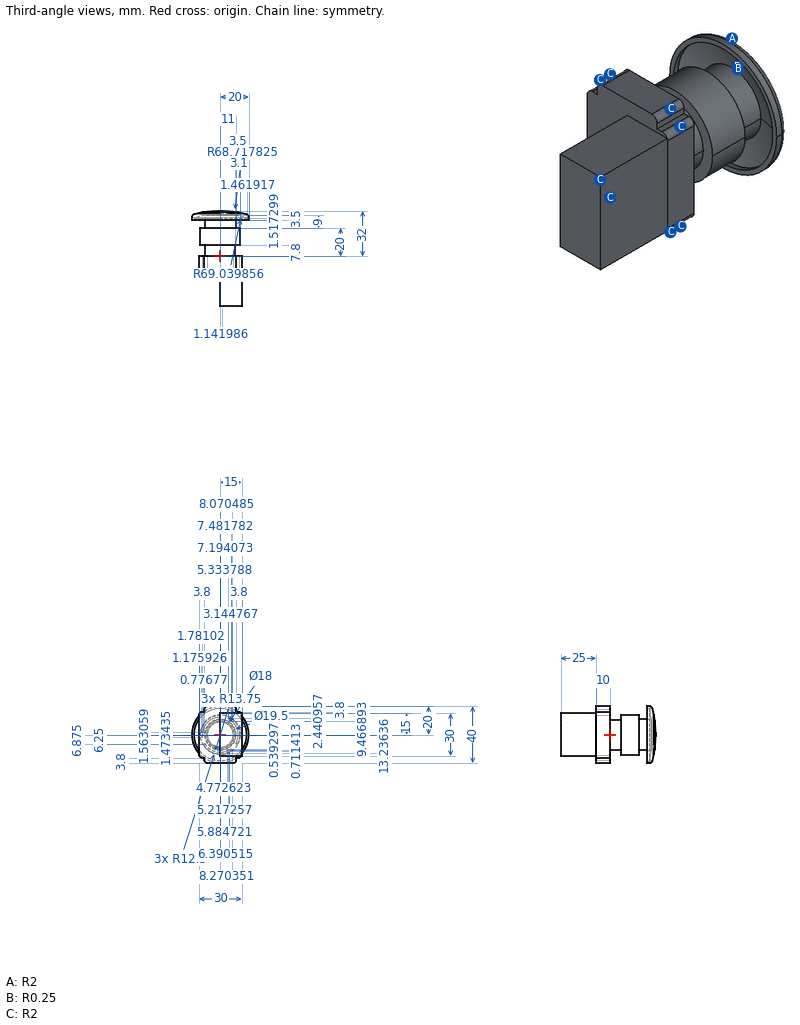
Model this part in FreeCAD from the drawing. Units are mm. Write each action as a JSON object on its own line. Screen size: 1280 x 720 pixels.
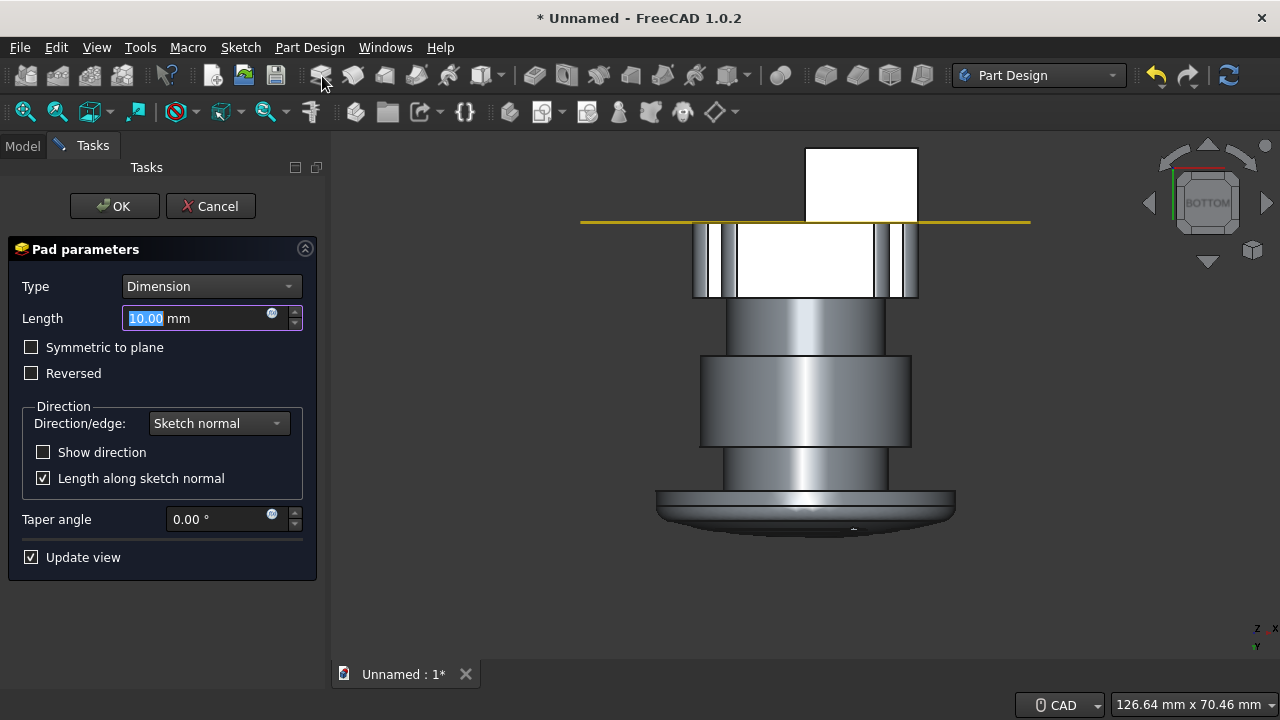
{"action": "type", "text": "25"}
{"action": "key", "text": "Tab"}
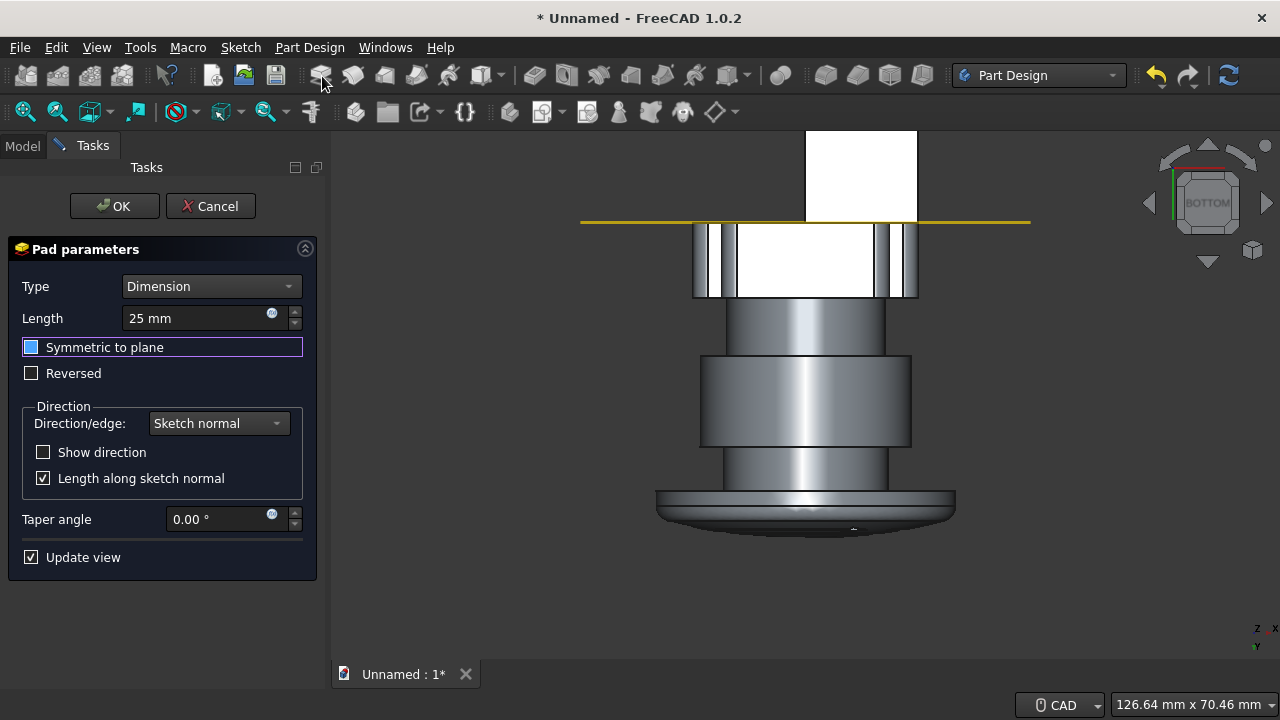
{"action": "left_click", "coordinate": [115, 206]}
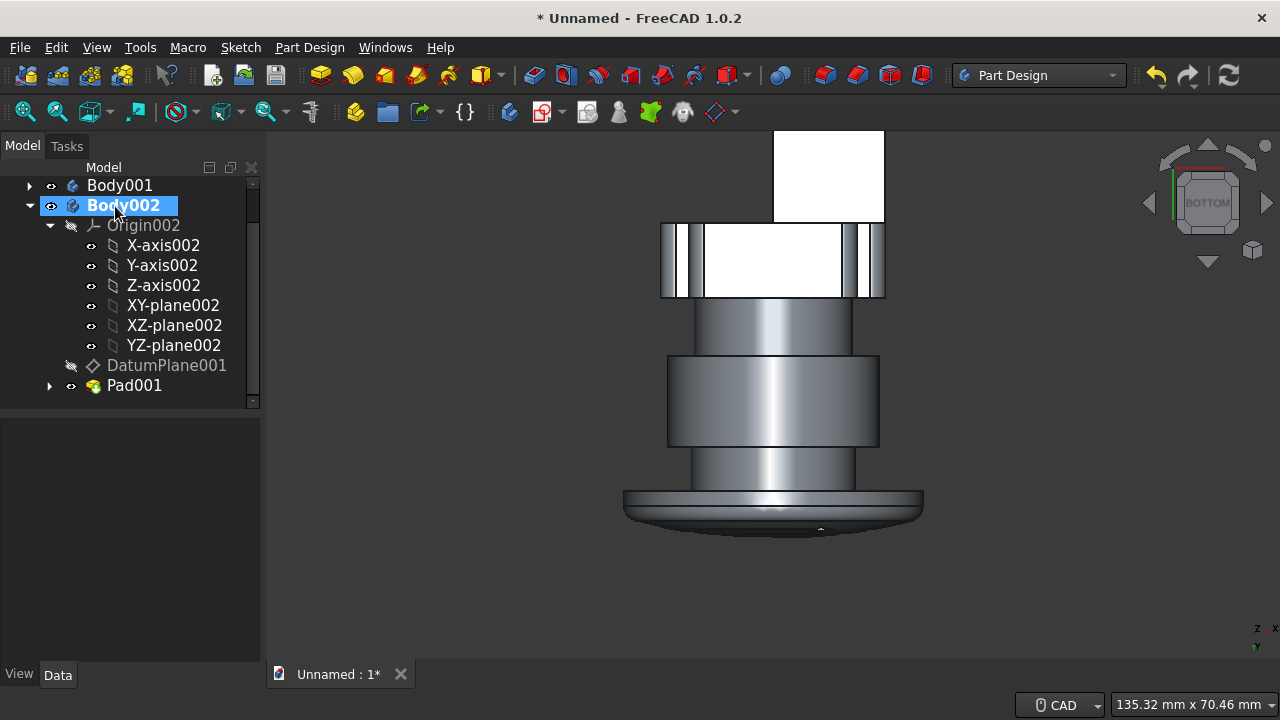
{"action": "key", "text": "0"}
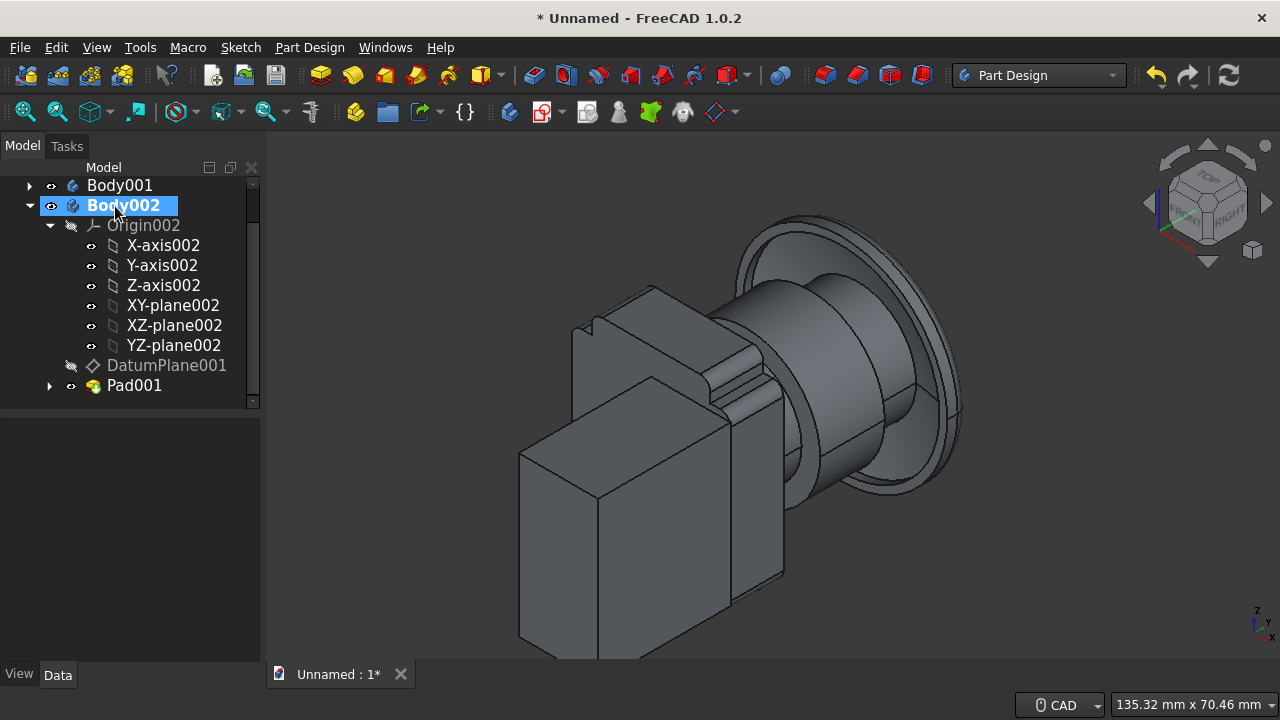
{"action": "left_click", "coordinate": [26, 112]}